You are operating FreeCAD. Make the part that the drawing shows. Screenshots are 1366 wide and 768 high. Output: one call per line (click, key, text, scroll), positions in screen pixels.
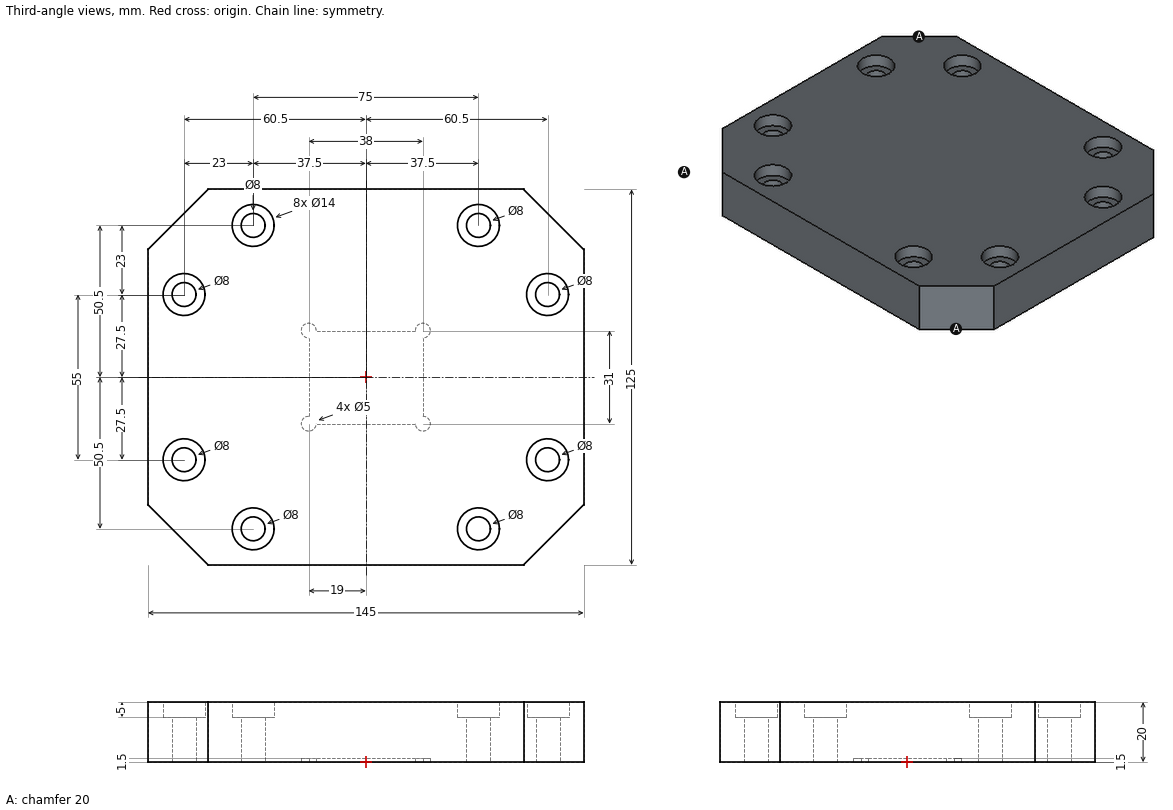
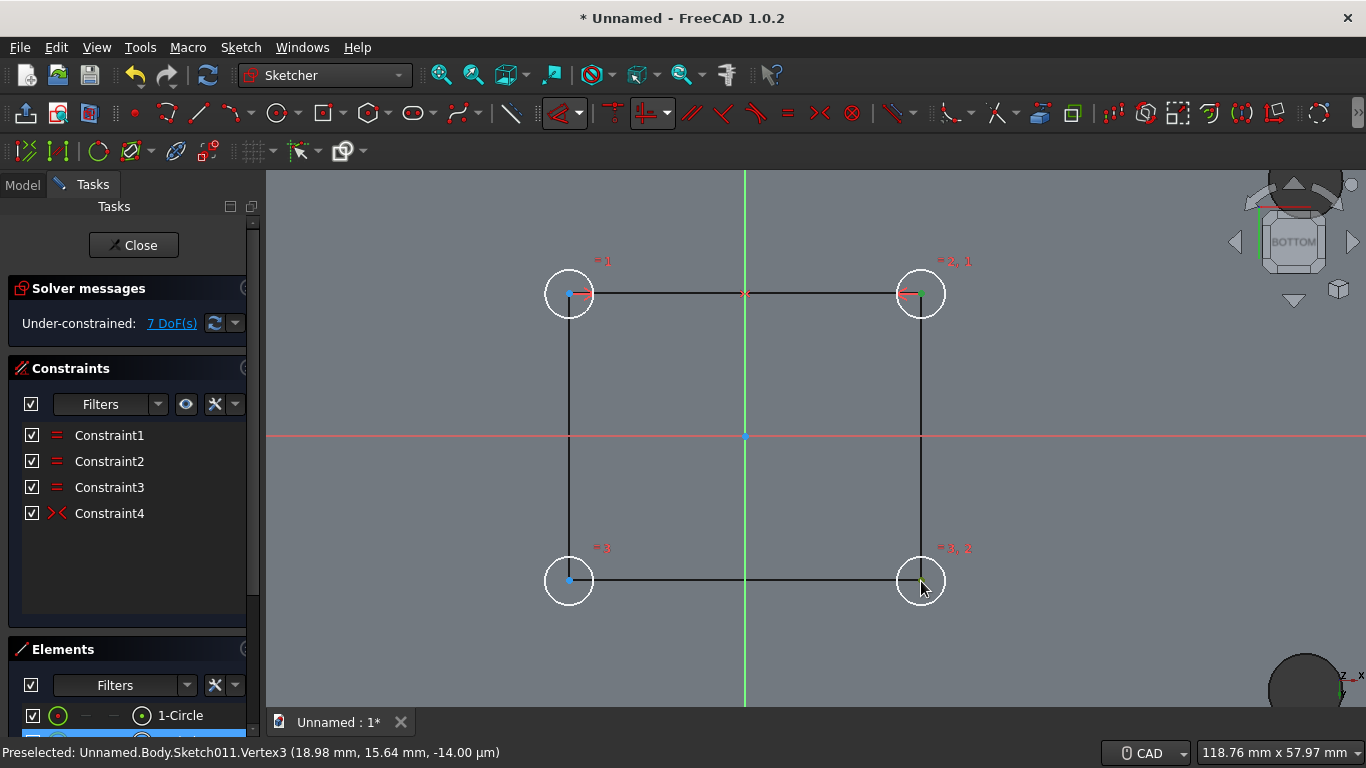
click(359, 436)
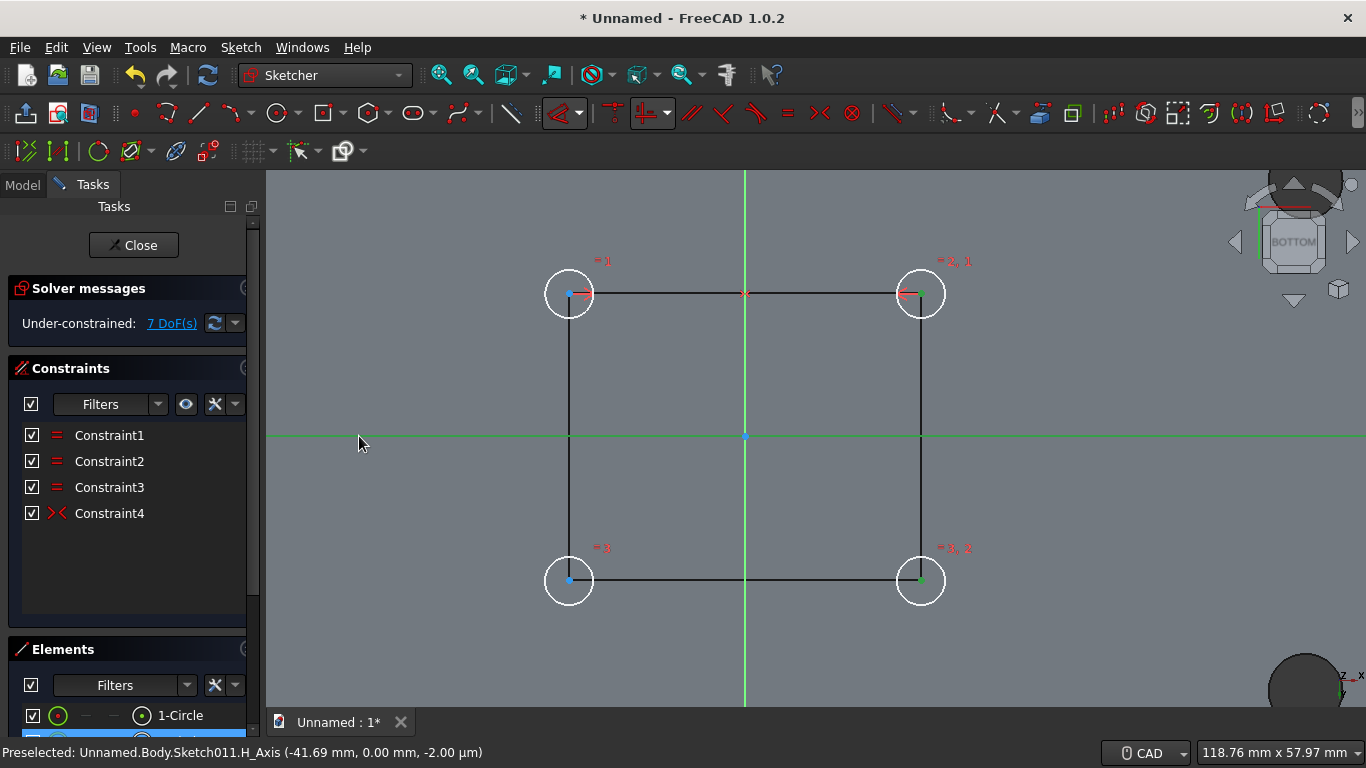
key(s)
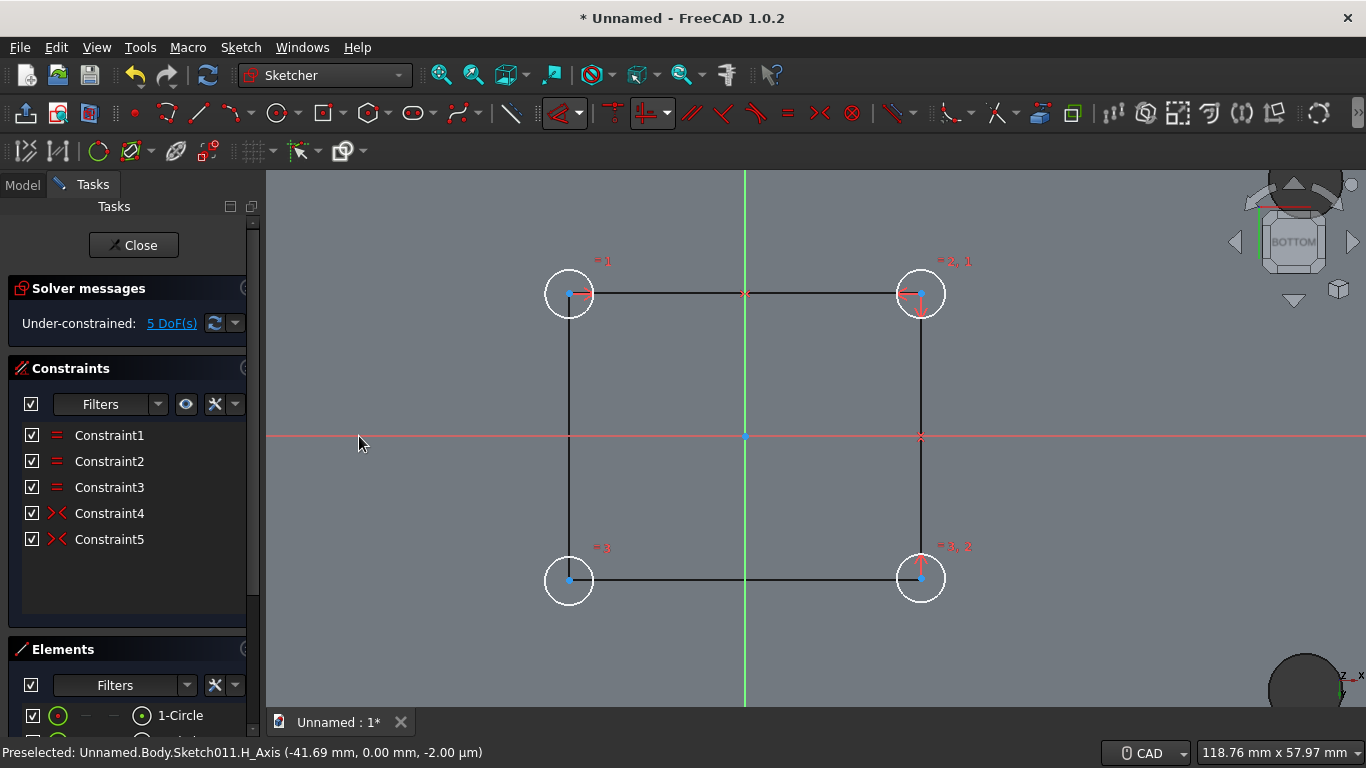
click(569, 294)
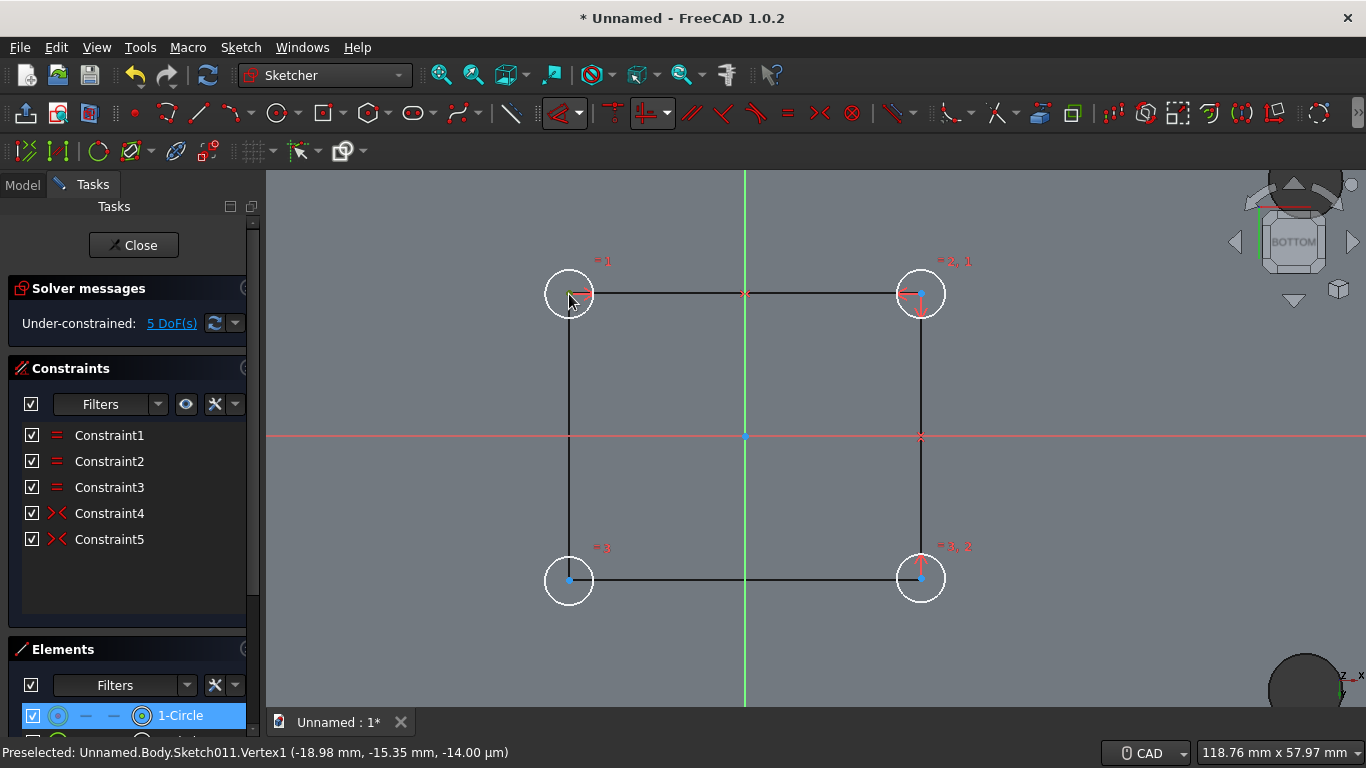
click(569, 581)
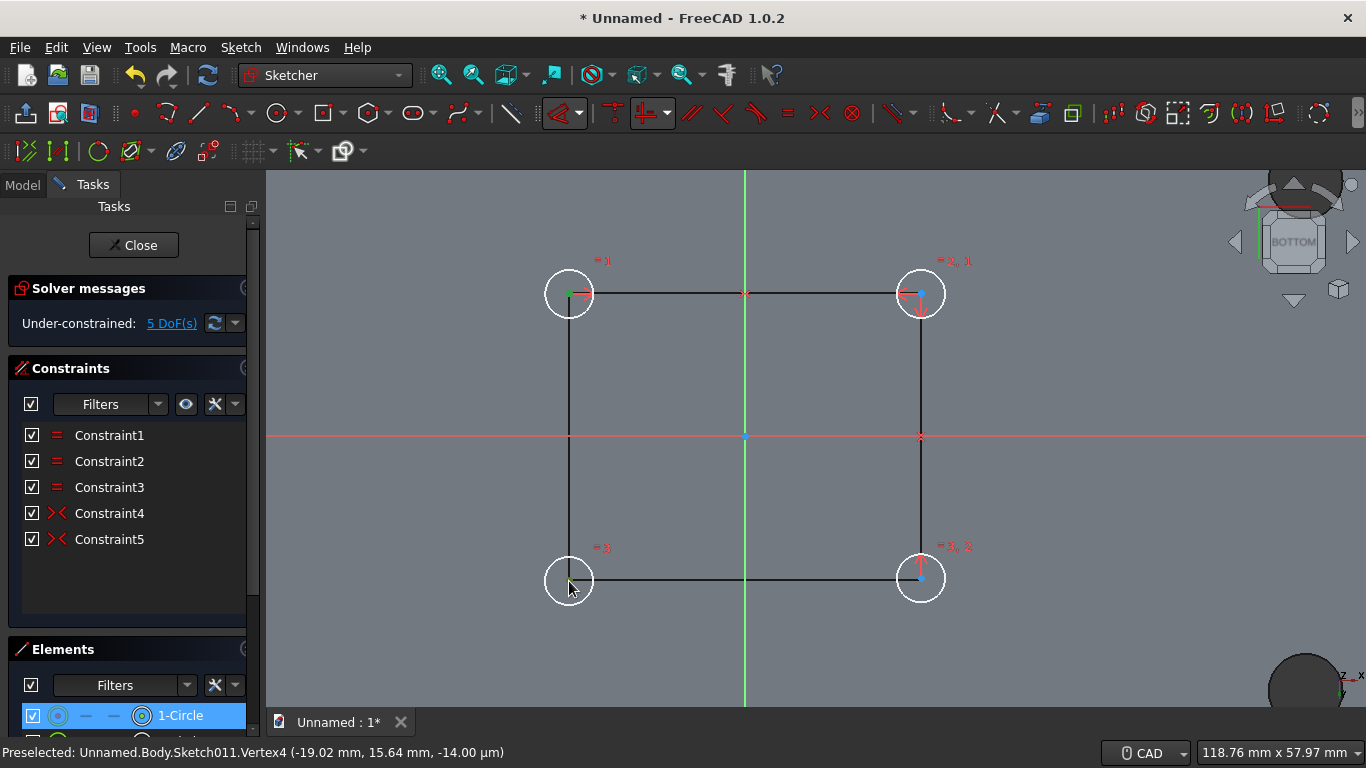
click(359, 436)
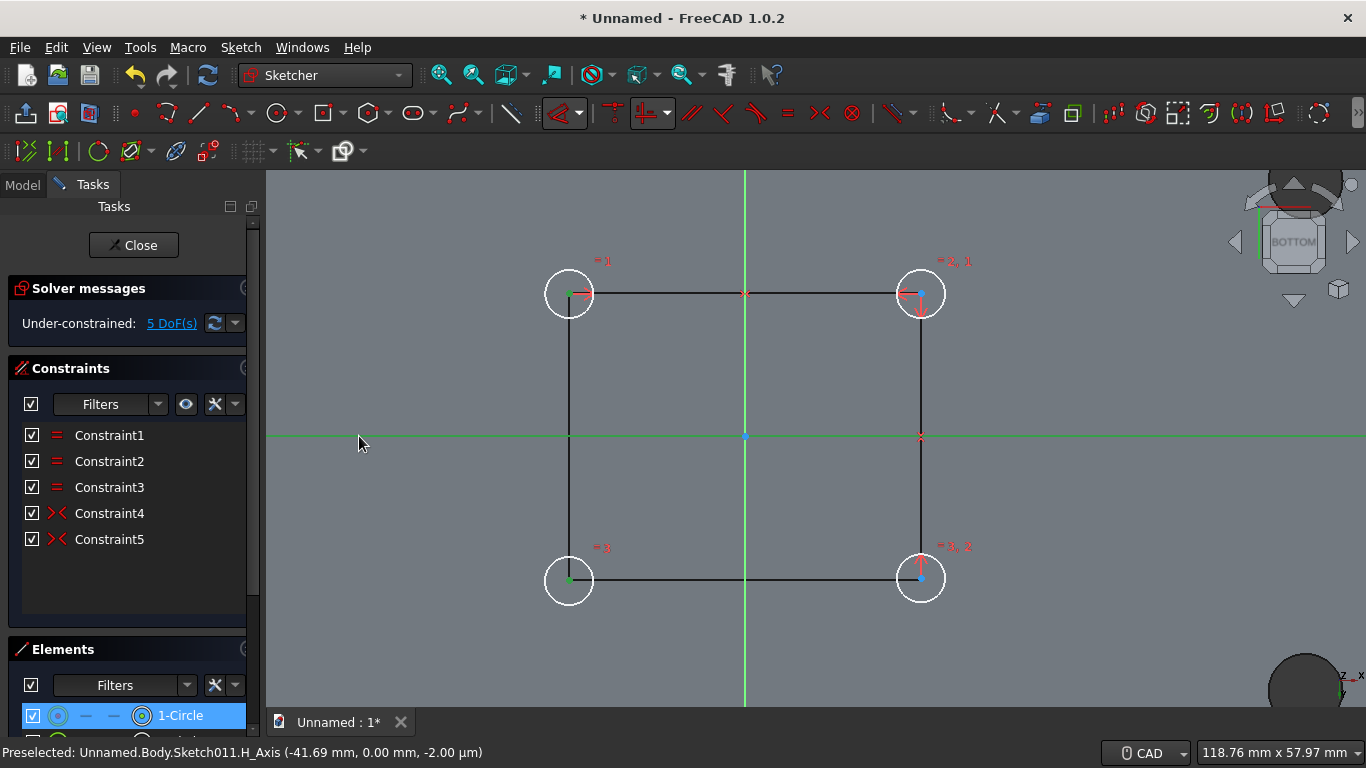
key(s)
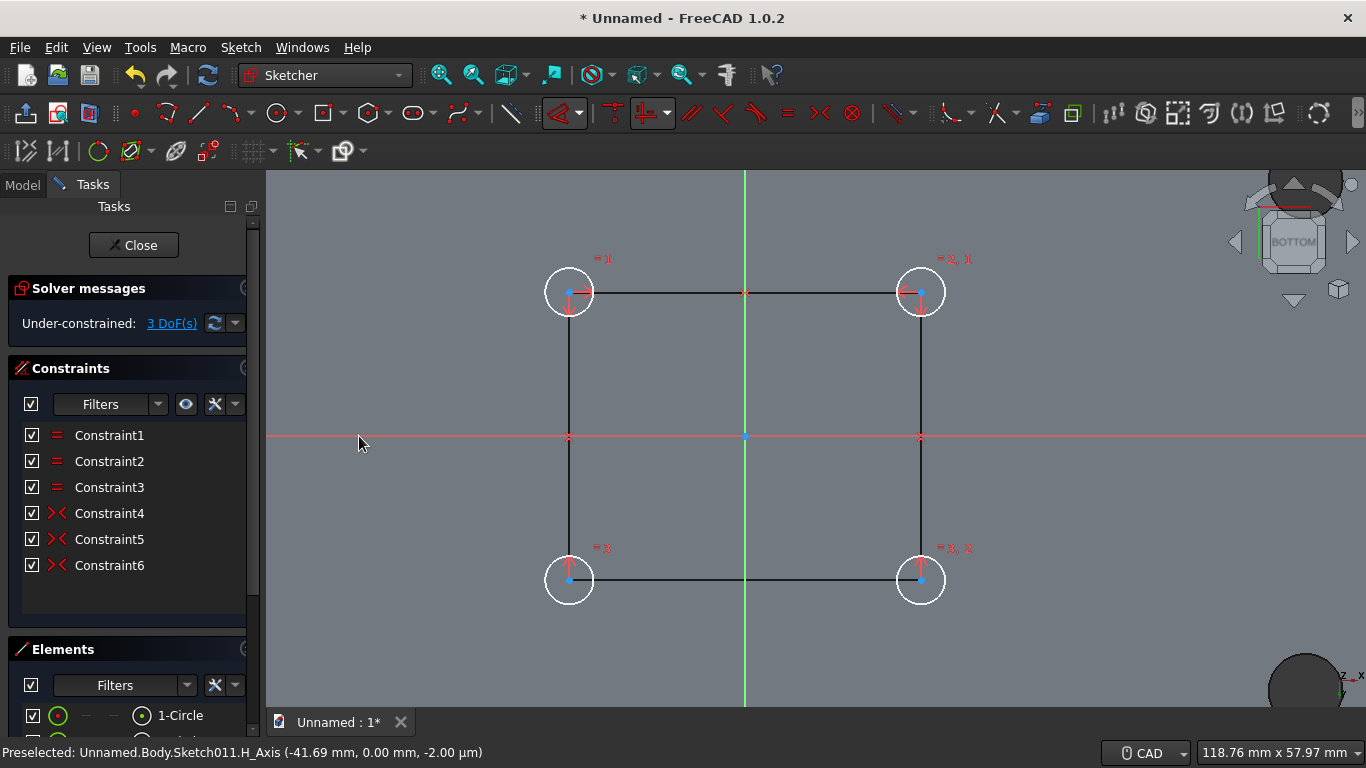
click(586, 275)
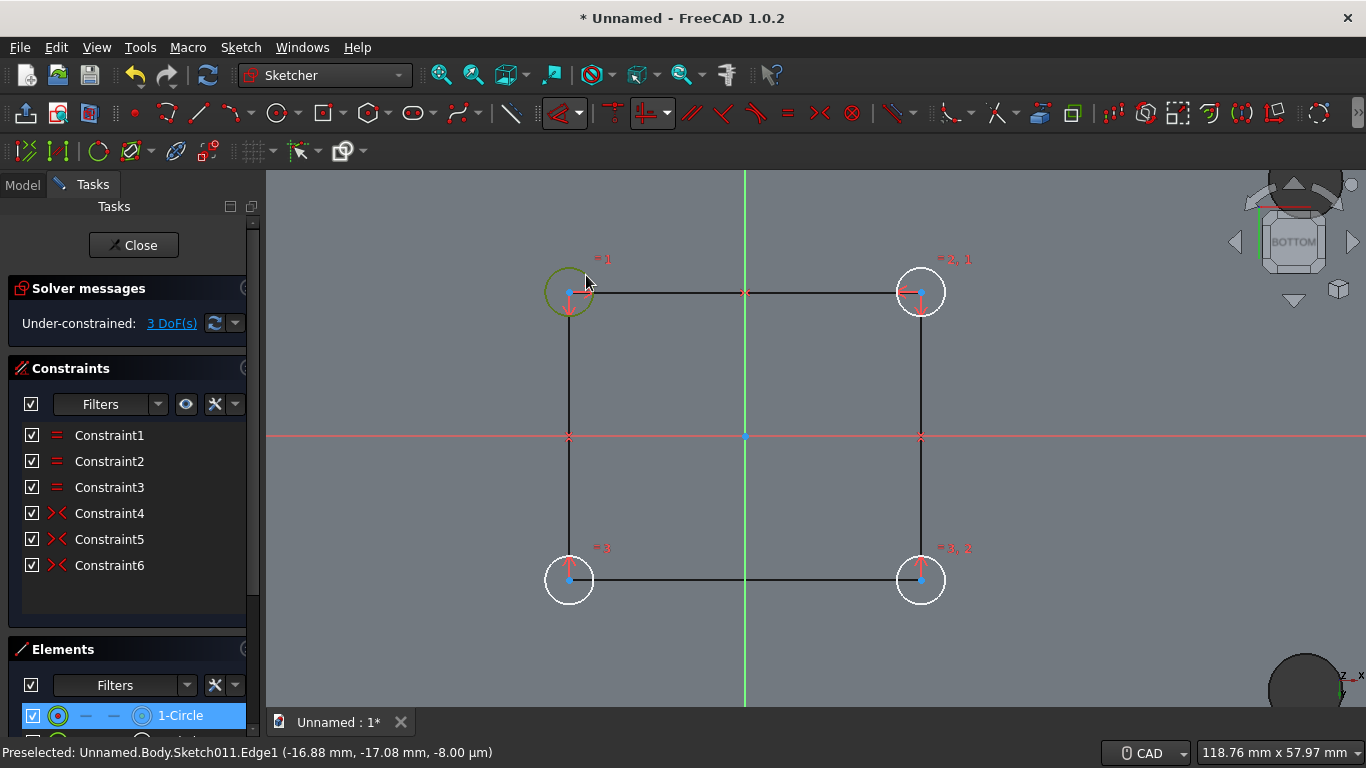
key(k)
key(o)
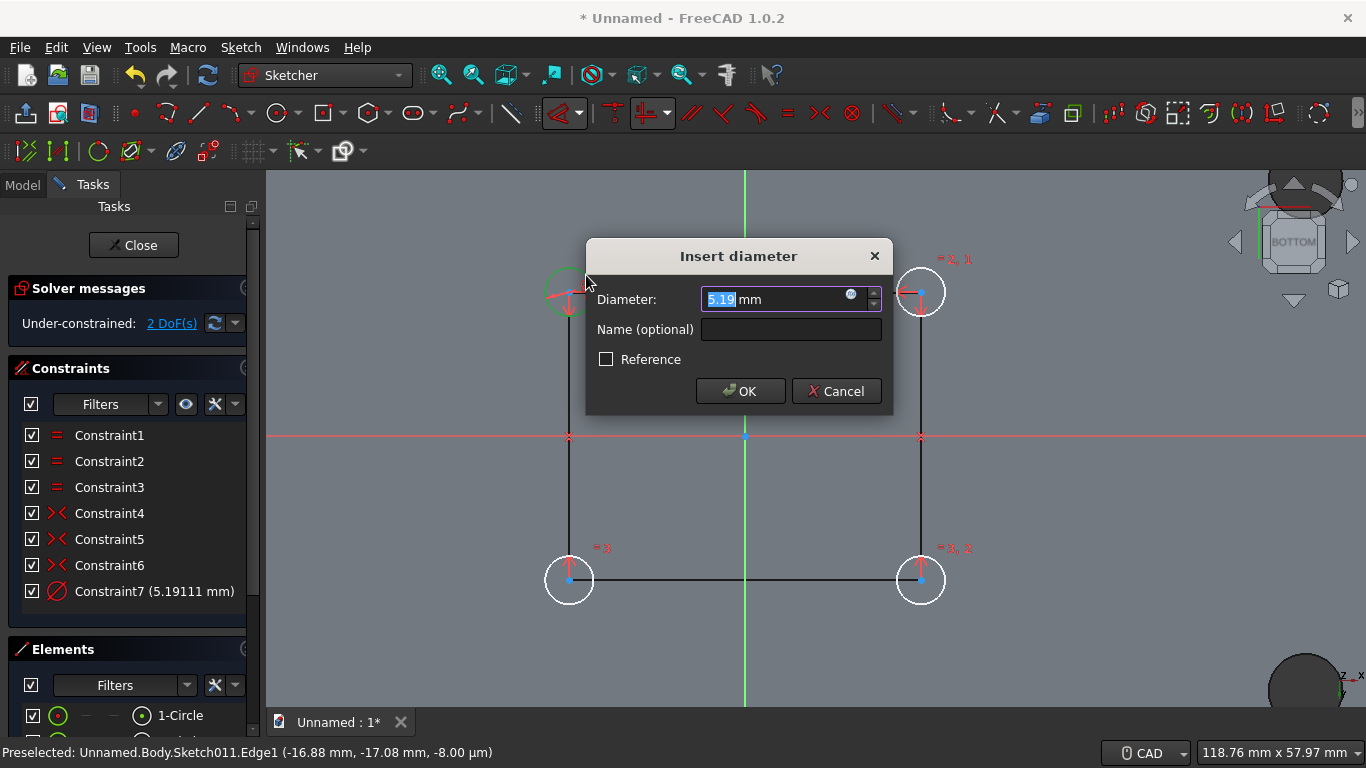
text(5)
key(Return)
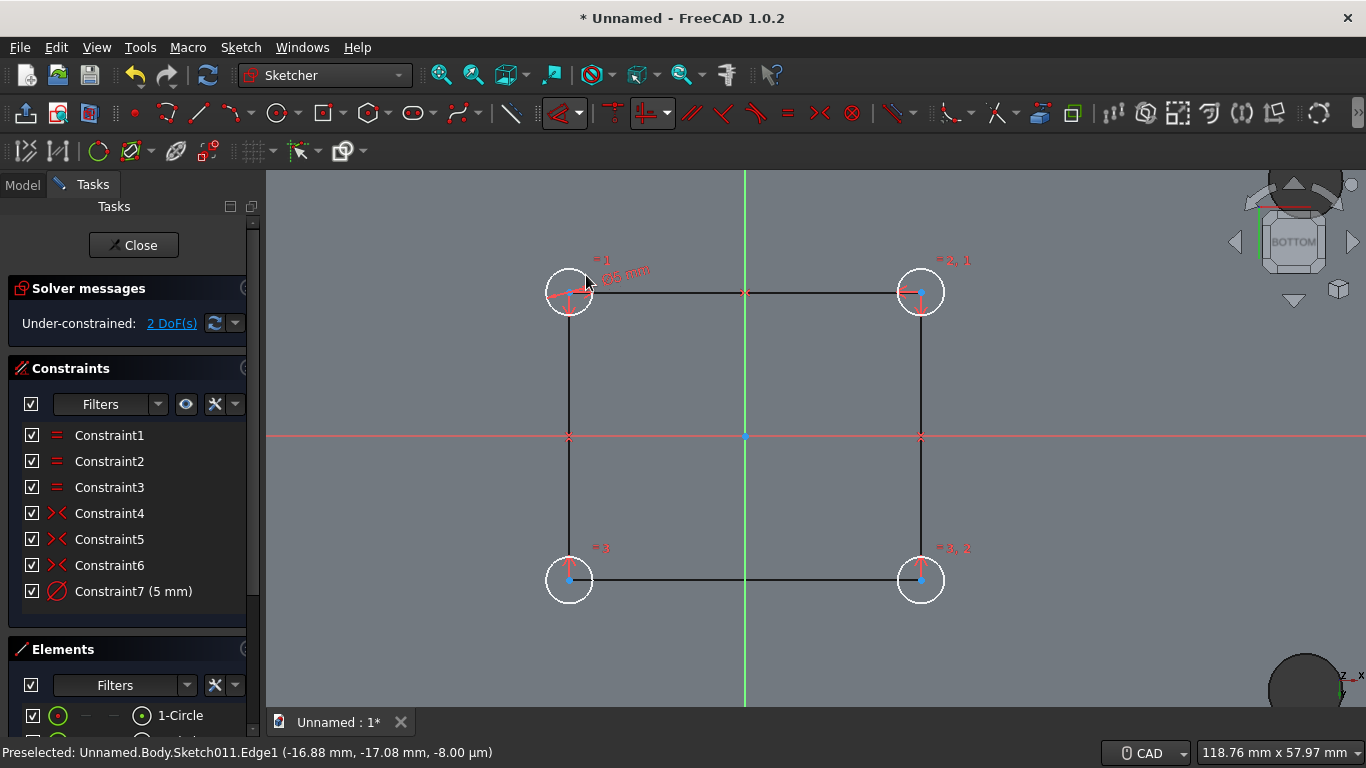
click(569, 292)